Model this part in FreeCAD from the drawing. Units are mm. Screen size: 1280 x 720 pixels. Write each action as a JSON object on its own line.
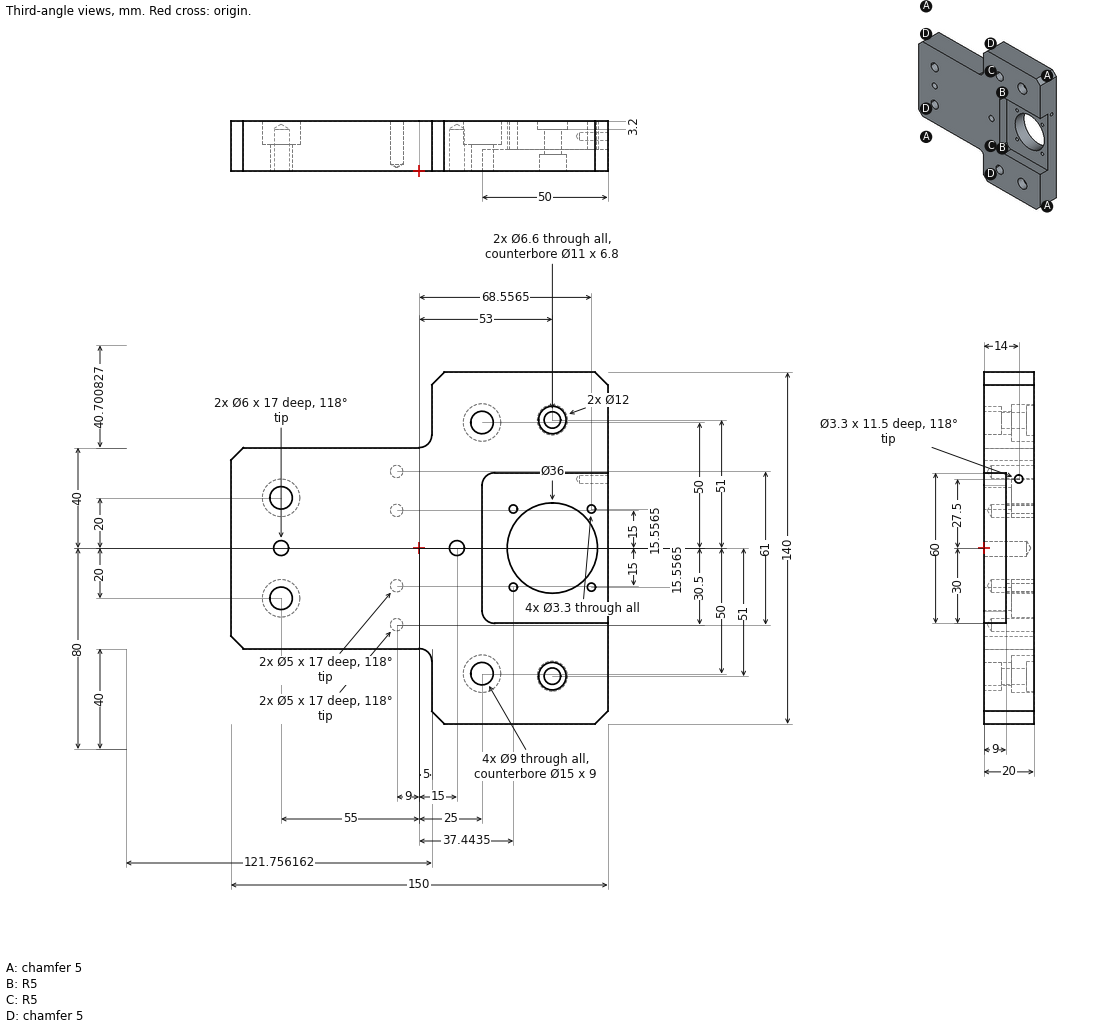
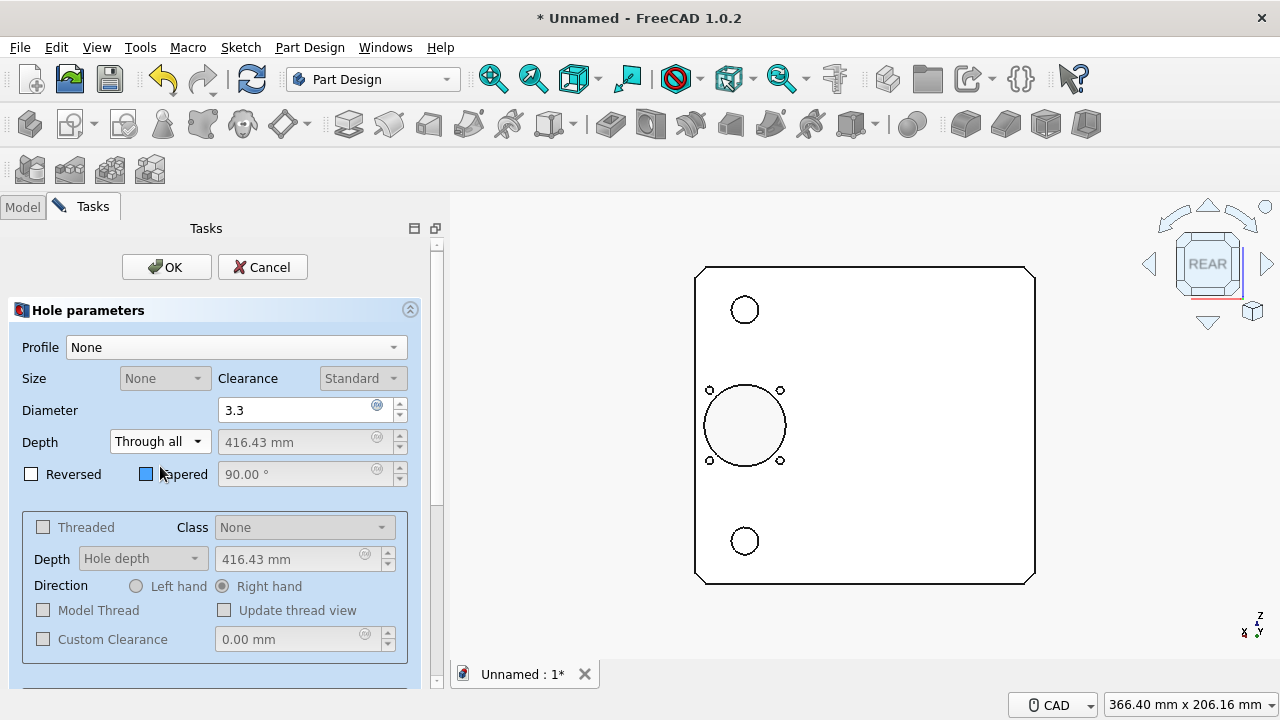
{"action": "left_click", "coordinate": [167, 267]}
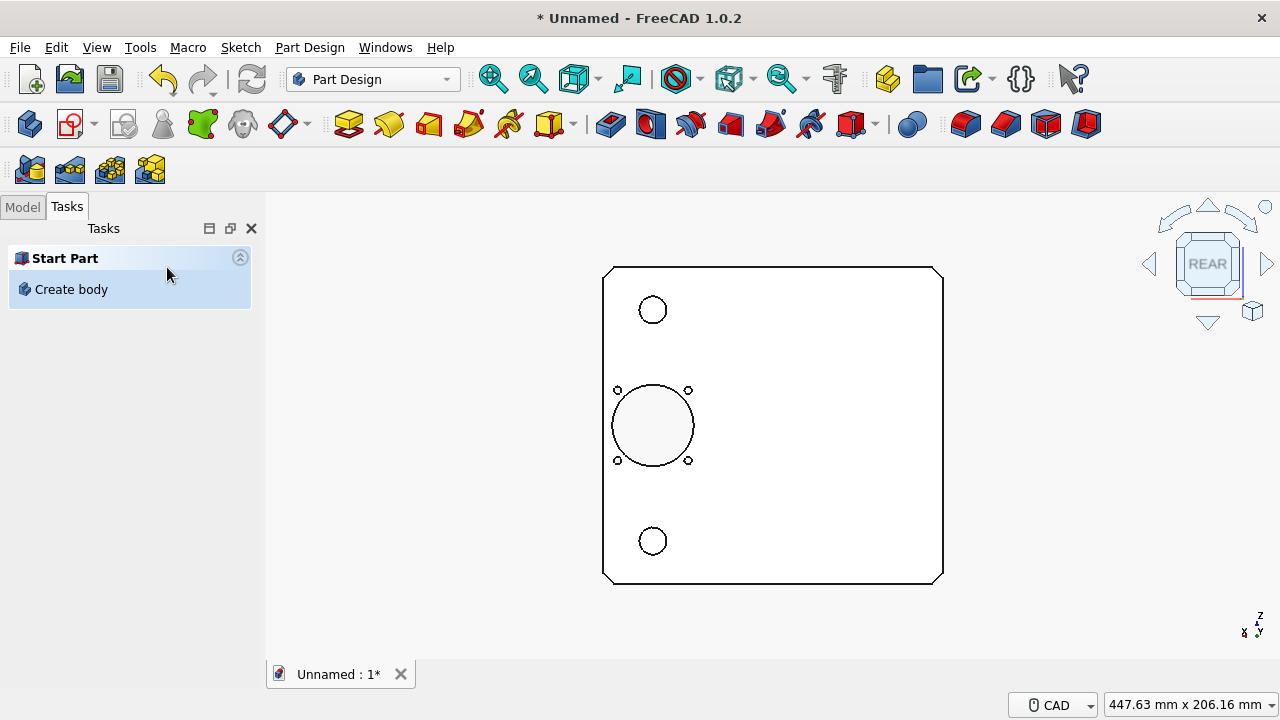
{"action": "key", "text": "0"}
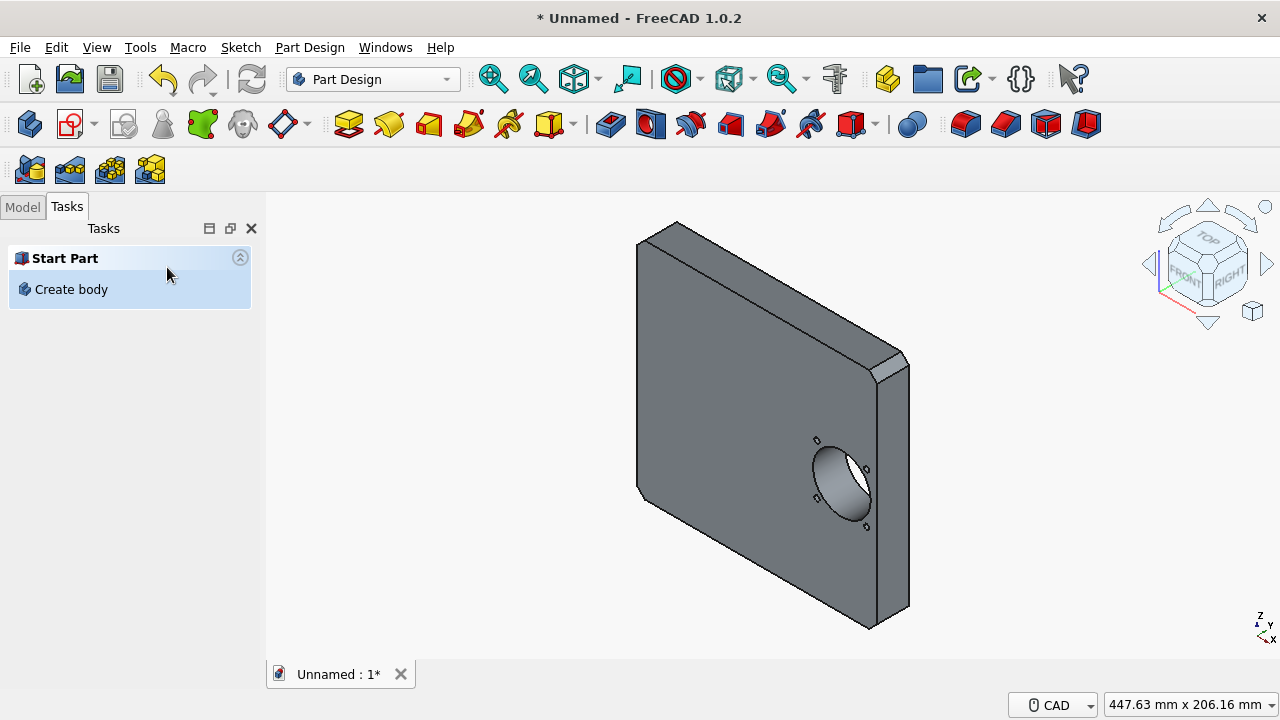
{"action": "left_click", "coordinate": [893, 425]}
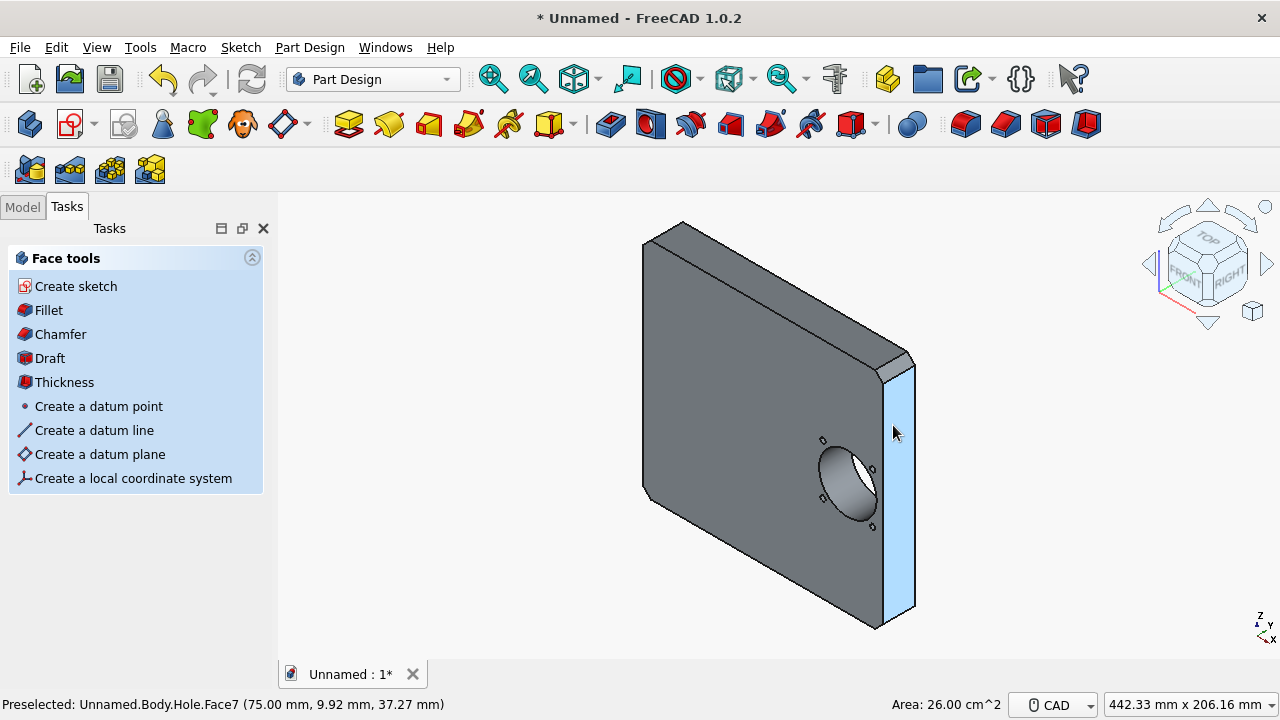
{"action": "left_click", "coordinate": [70, 124]}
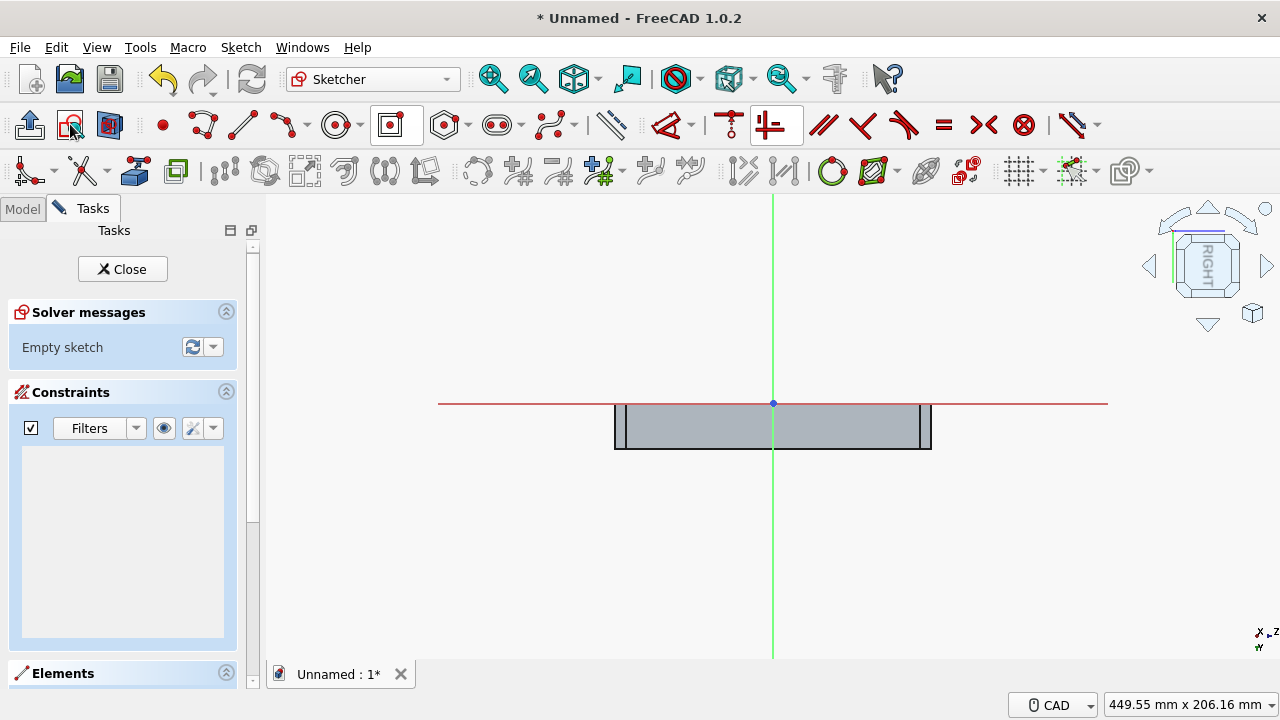
{"action": "scroll", "coordinate": [795, 410], "scroll_direction": "up", "scroll_amount": 7}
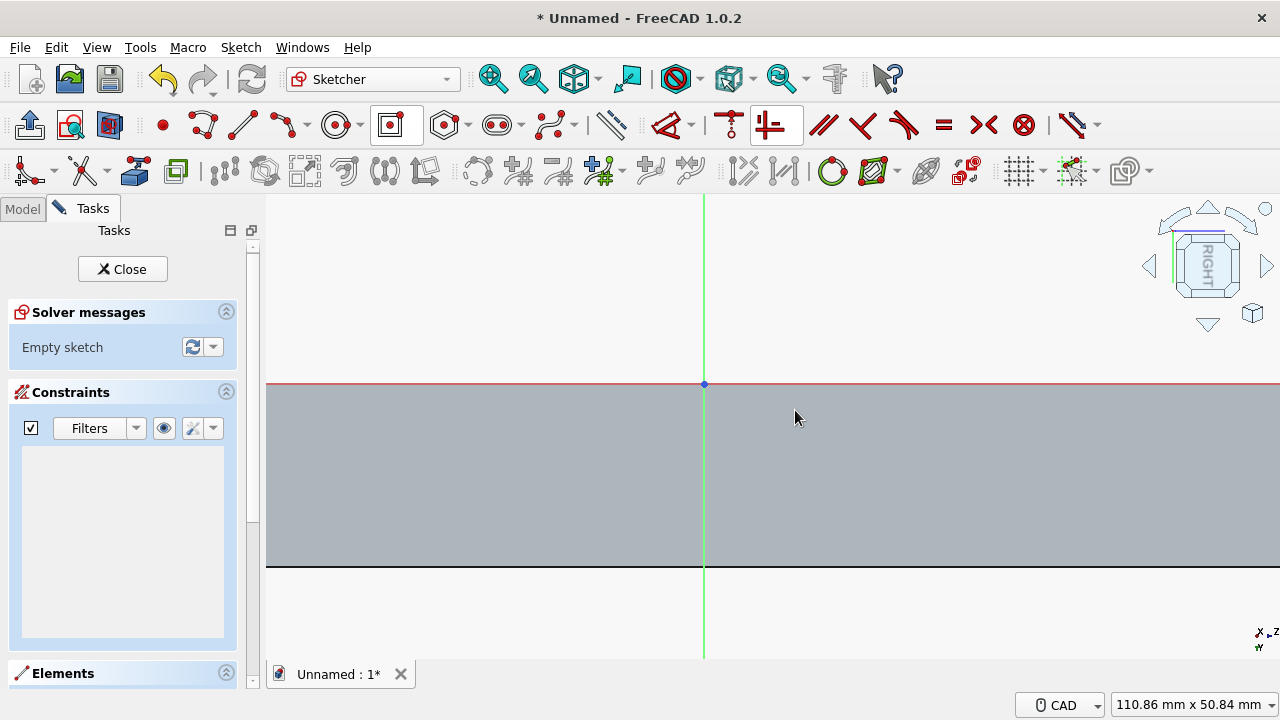
{"action": "left_click", "coordinate": [418, 126]}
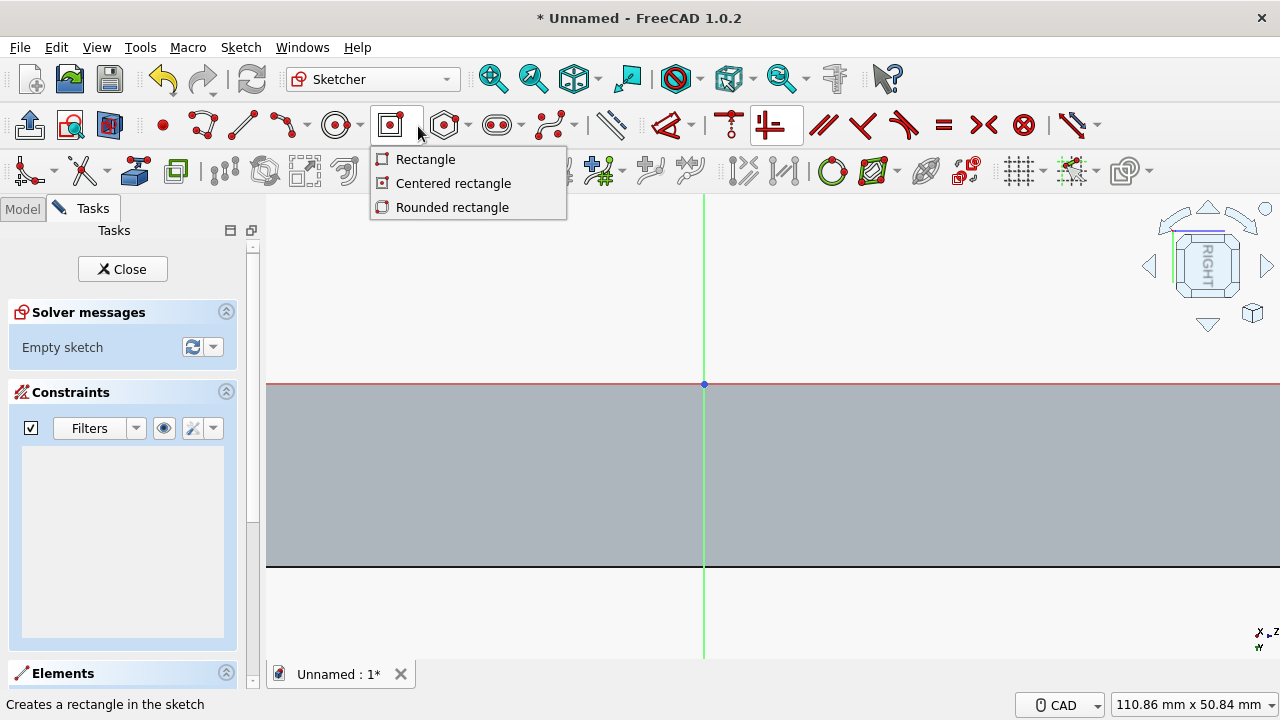
{"action": "left_click", "coordinate": [468, 159]}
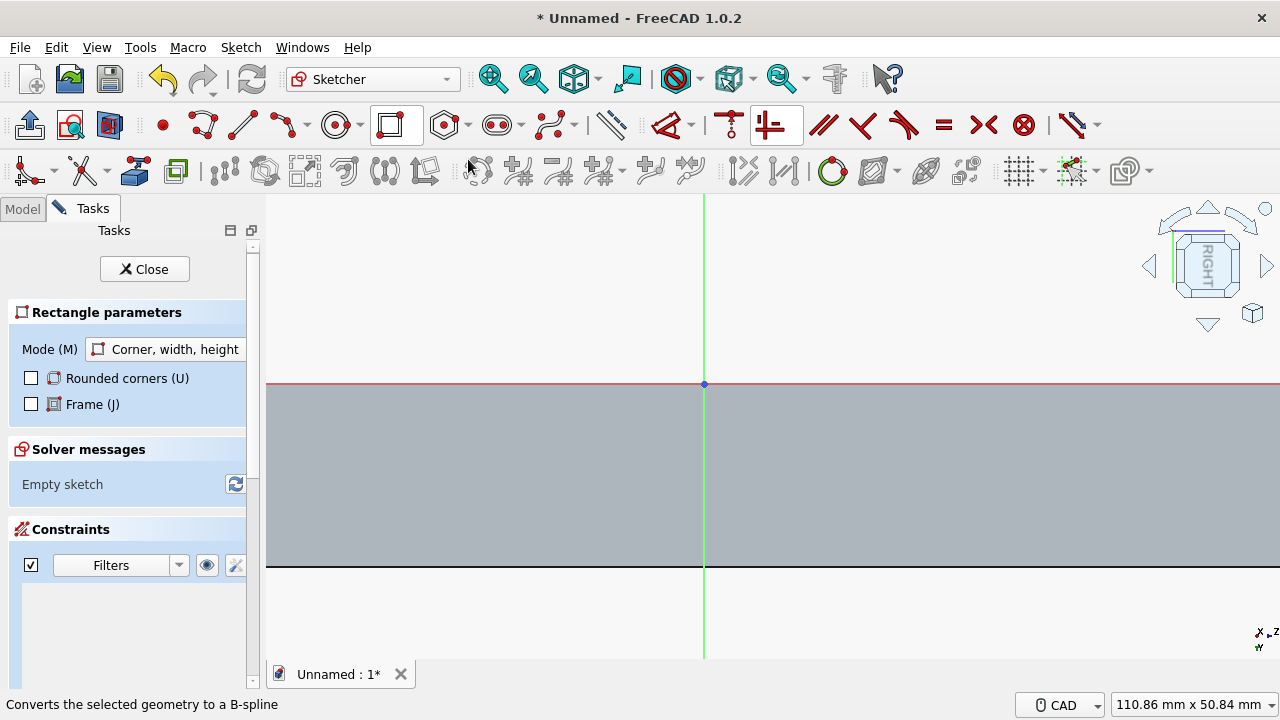
{"action": "left_click", "coordinate": [430, 384]}
{"action": "left_click", "coordinate": [979, 466]}
{"action": "key", "text": "Escape"}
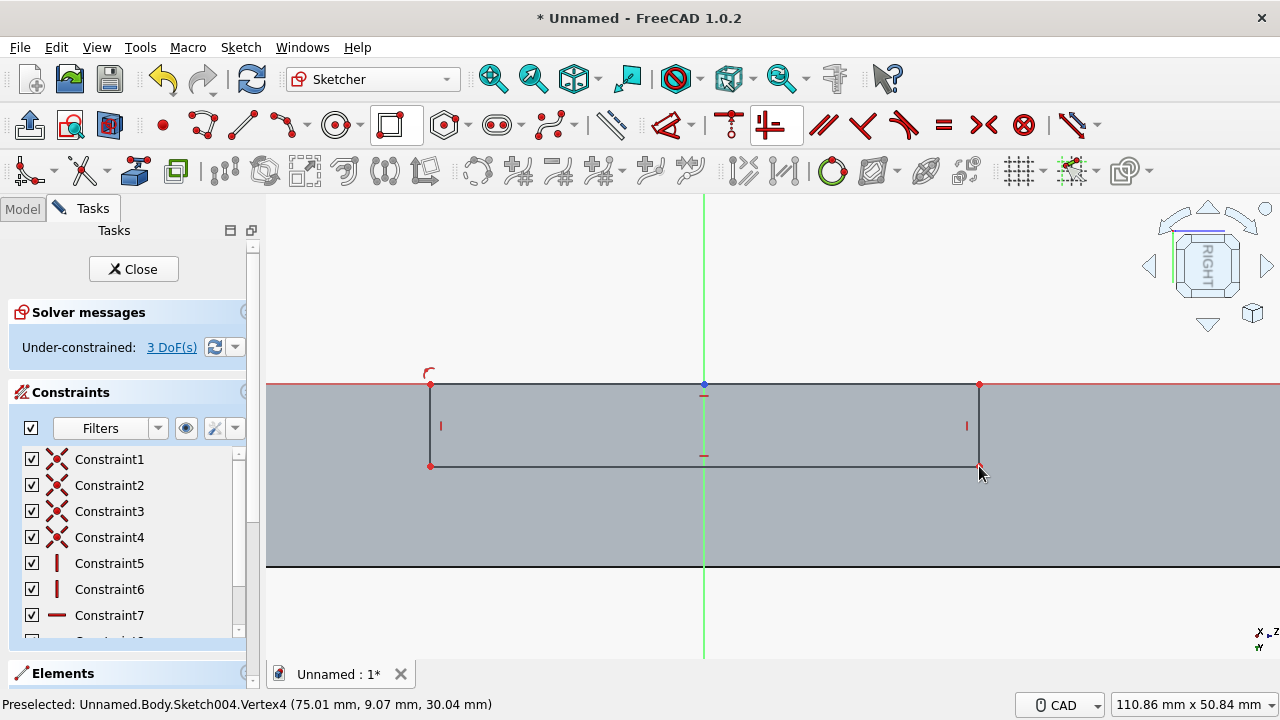
{"action": "left_click", "coordinate": [666, 126]}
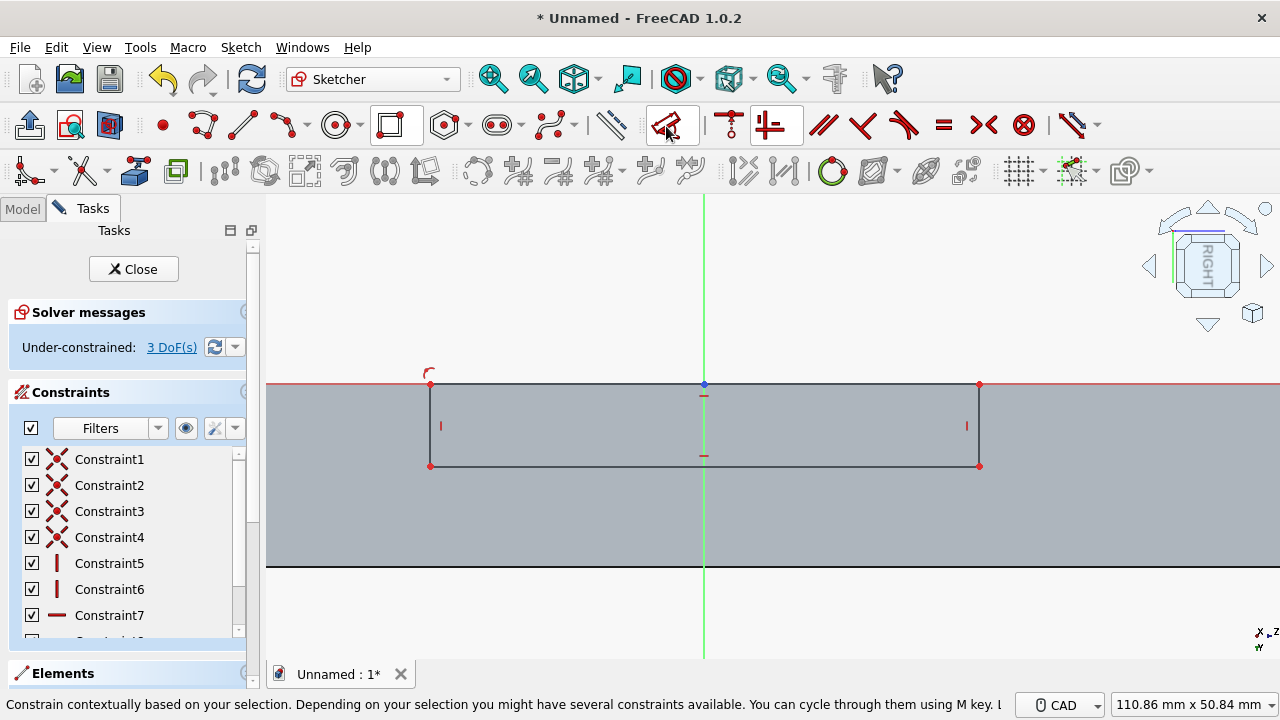
{"action": "left_click", "coordinate": [430, 409]}
{"action": "left_click", "coordinate": [396, 426]}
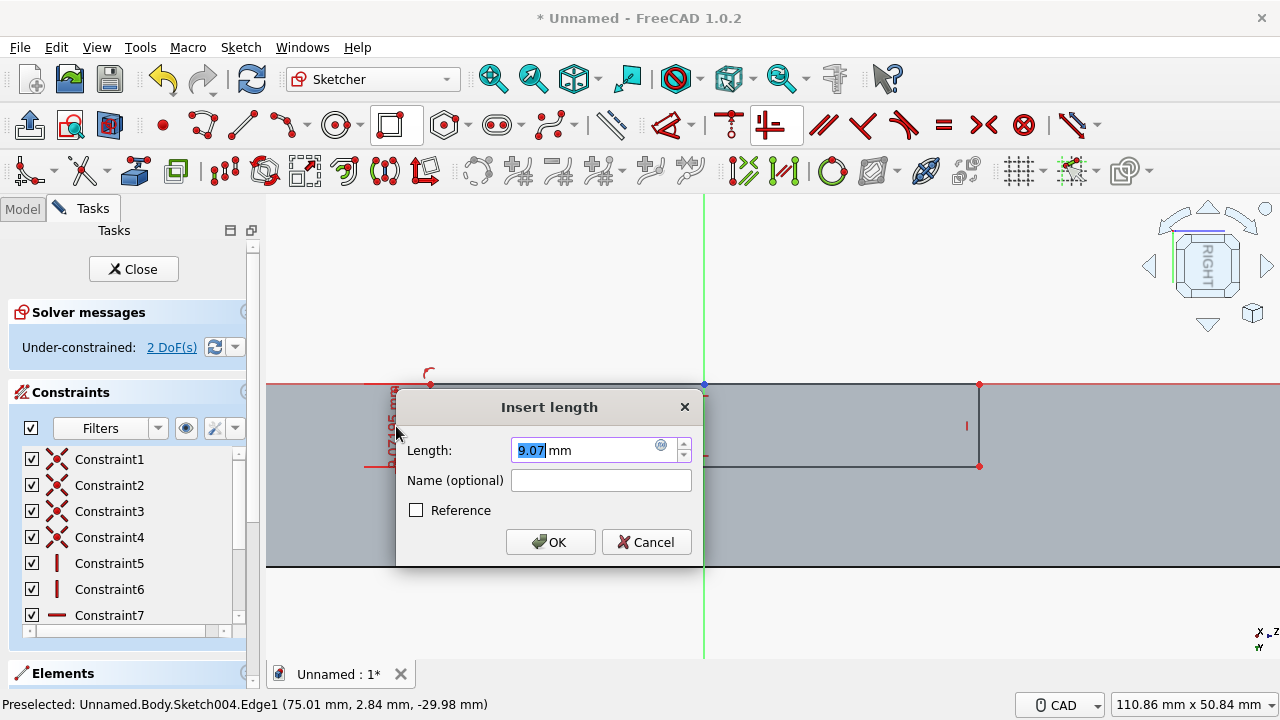
{"action": "type", "text": "9"}
{"action": "key", "text": "Return"}